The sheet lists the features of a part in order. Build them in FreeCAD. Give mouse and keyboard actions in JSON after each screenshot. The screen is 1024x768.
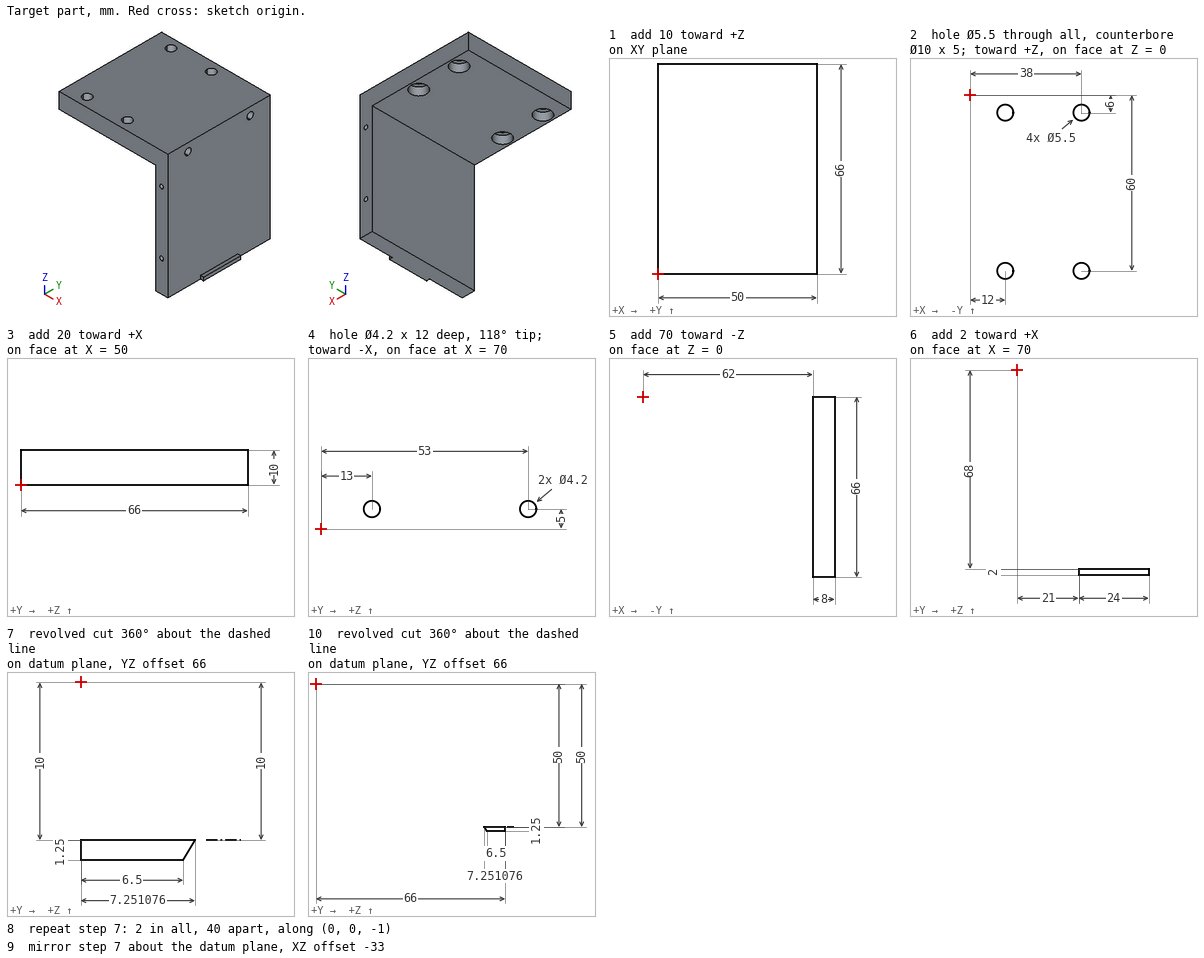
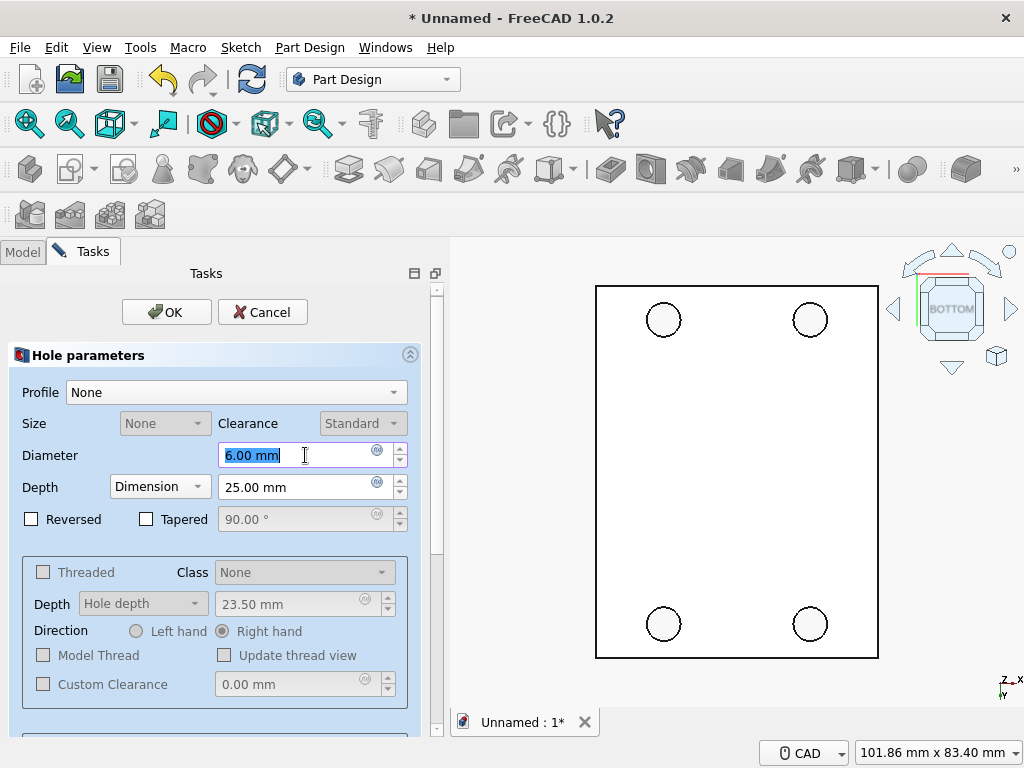
{"action": "type", "text": "5.5"}
{"action": "key", "text": "Tab"}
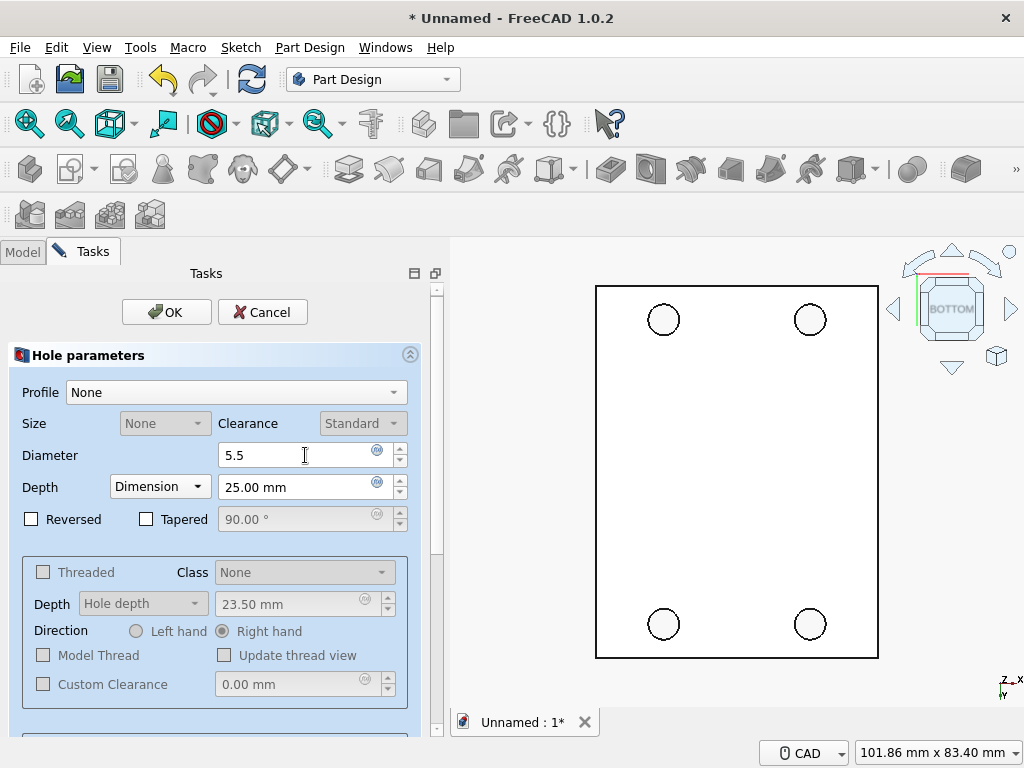
{"action": "left_click", "coordinate": [161, 486]}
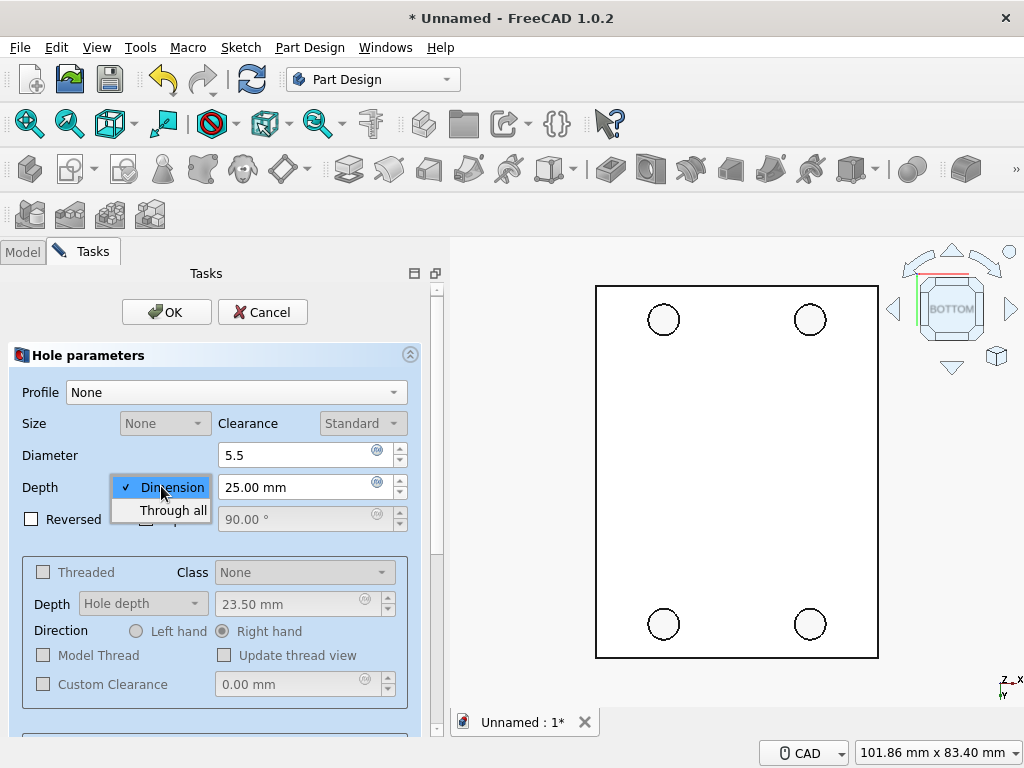
{"action": "left_click", "coordinate": [160, 510]}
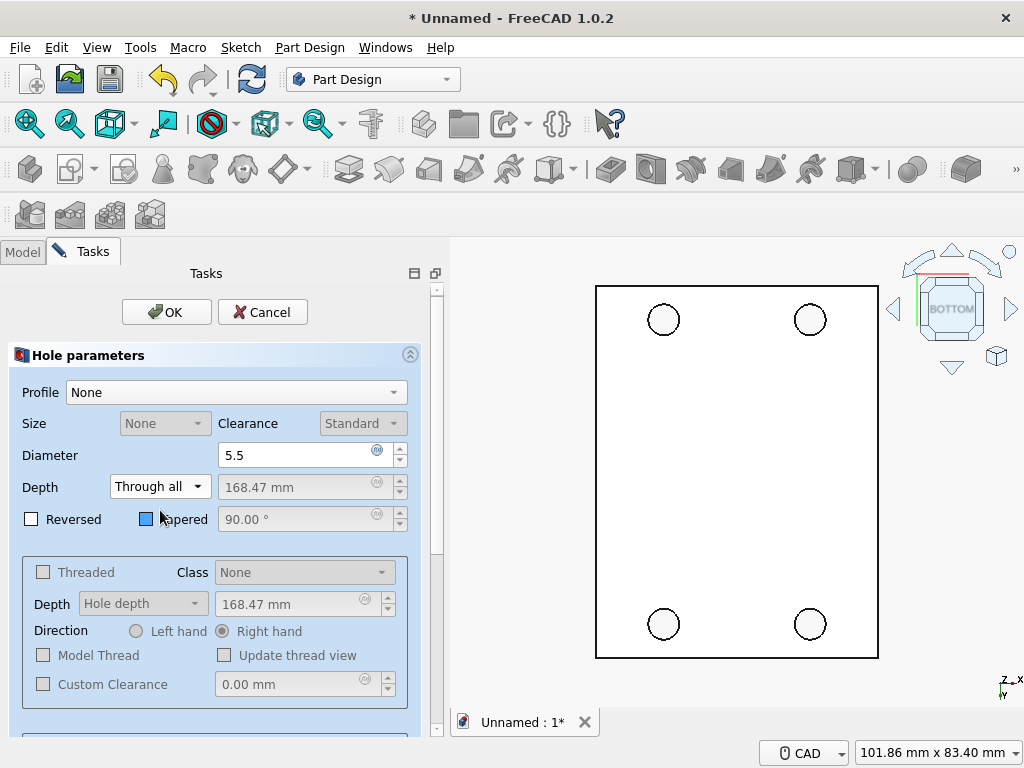
{"action": "scroll", "coordinate": [437, 510], "scroll_direction": "down", "scroll_amount": 2}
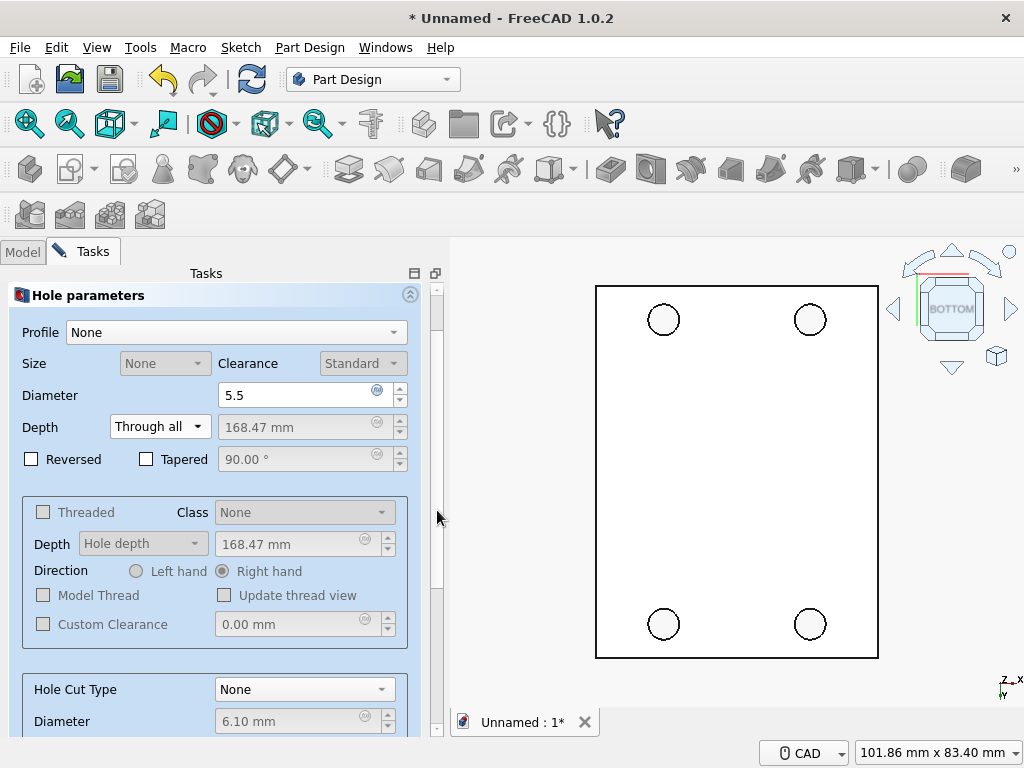
{"action": "left_click", "coordinate": [306, 630]}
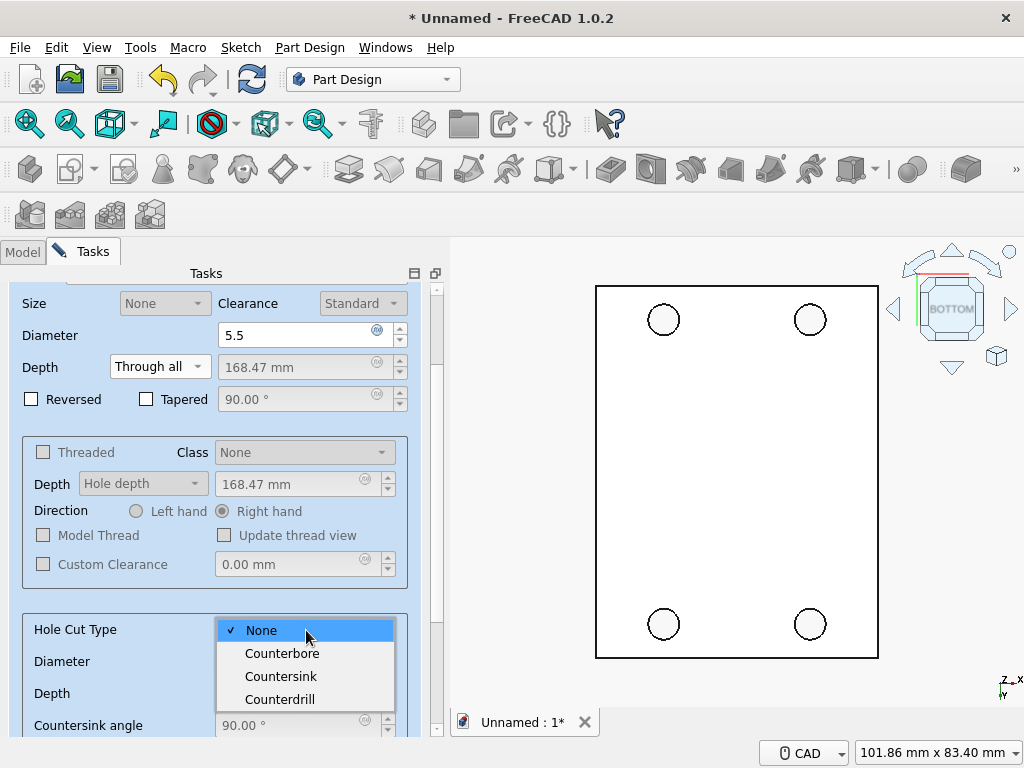
{"action": "left_click", "coordinate": [304, 654]}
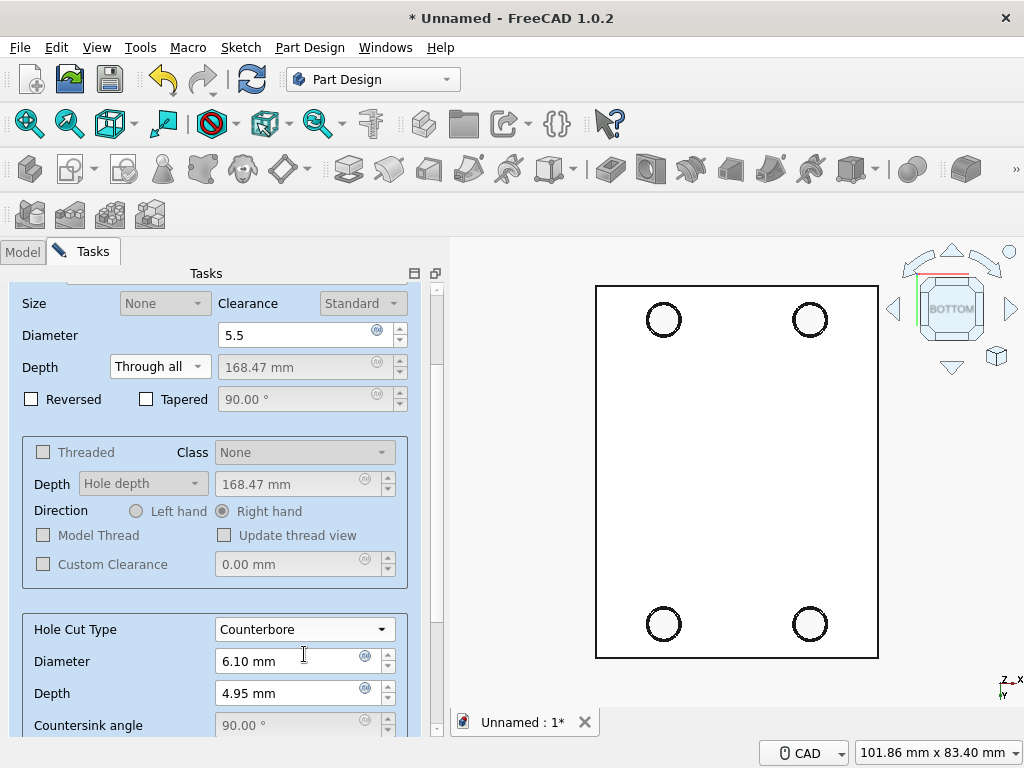
{"action": "triple_click", "coordinate": [298, 661]}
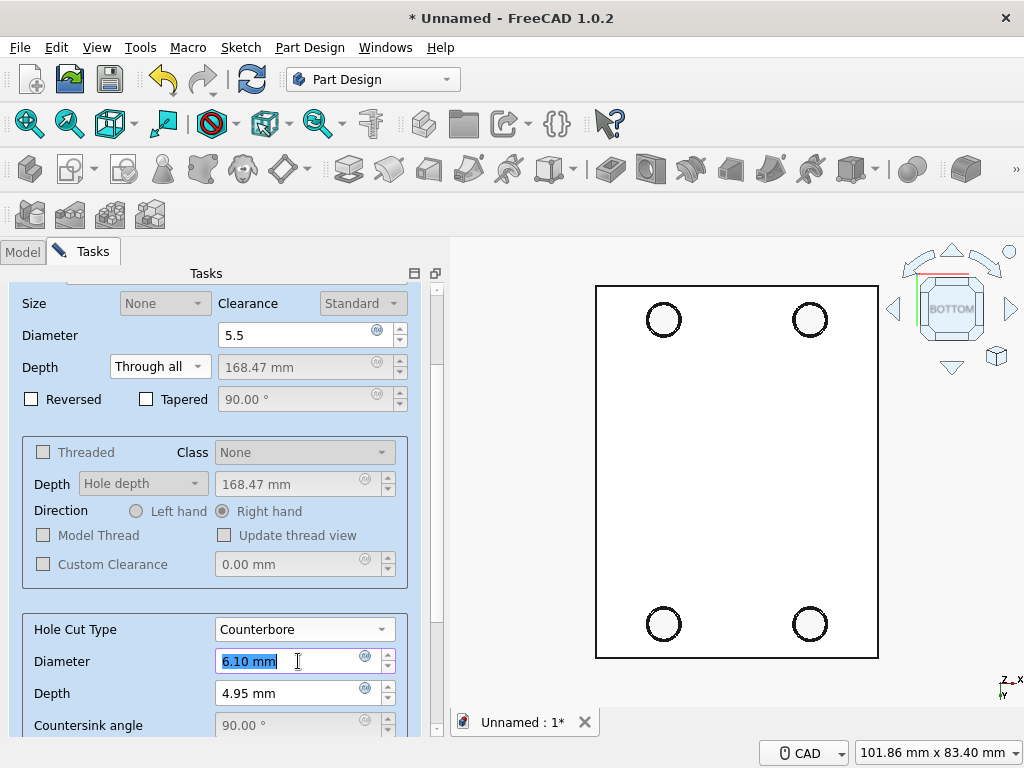
{"action": "type", "text": "10"}
{"action": "key", "text": "Tab"}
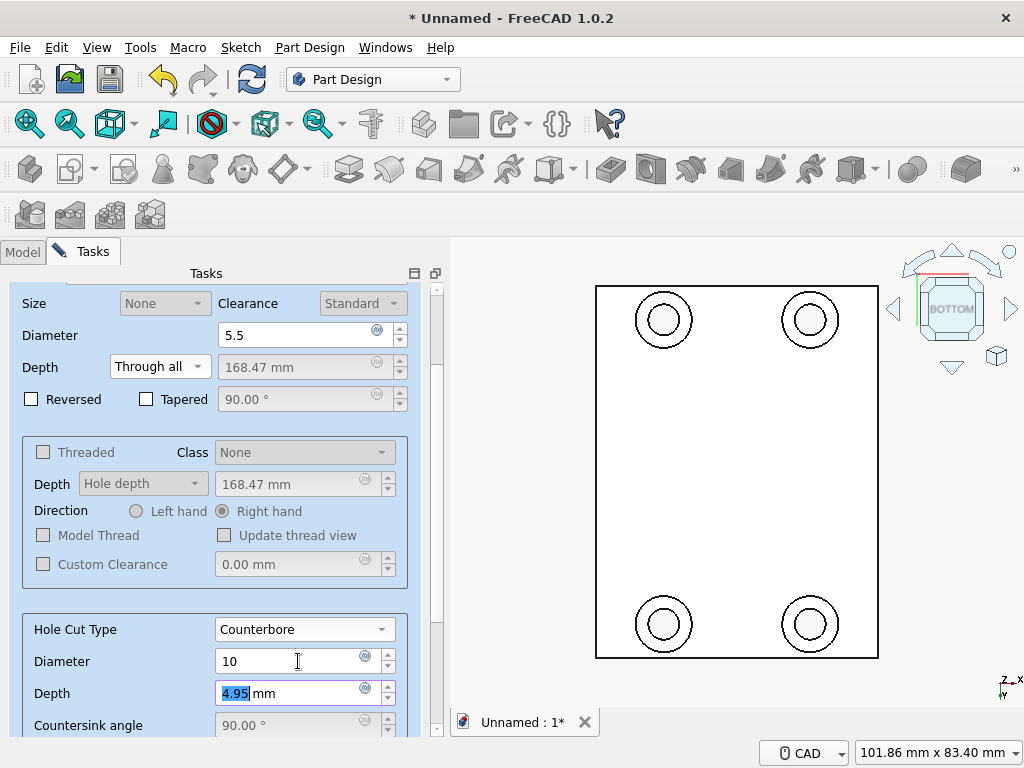
{"action": "type", "text": "5"}
{"action": "key", "text": "Tab"}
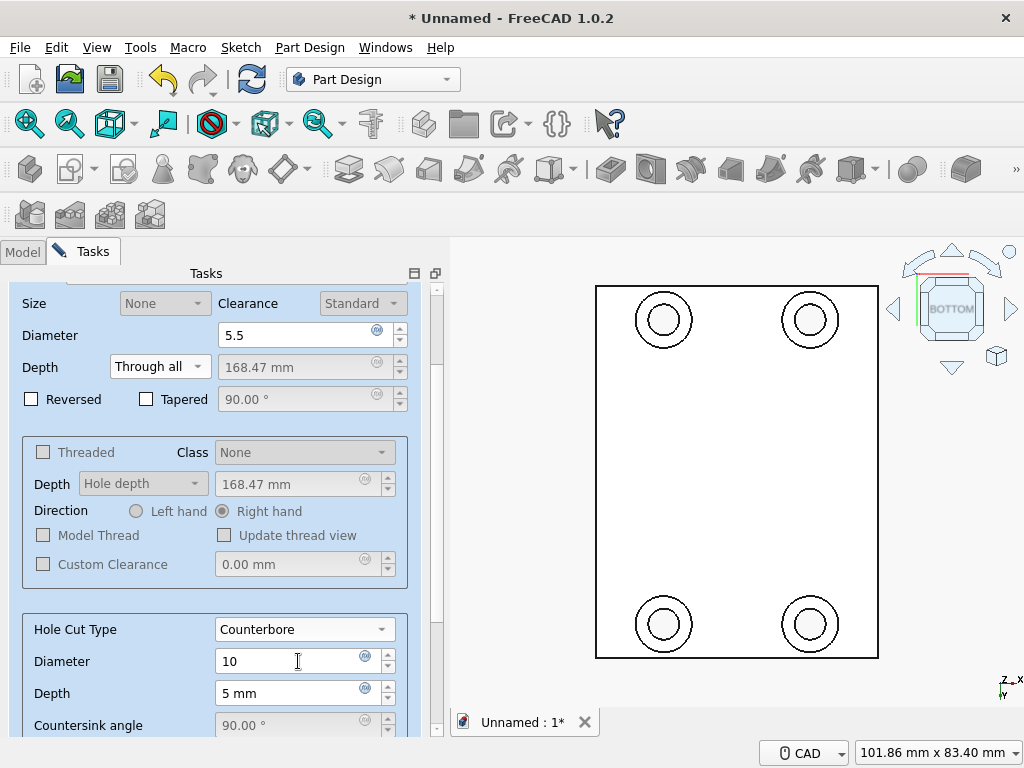
{"action": "scroll", "coordinate": [437, 510], "scroll_direction": "up", "scroll_amount": 3}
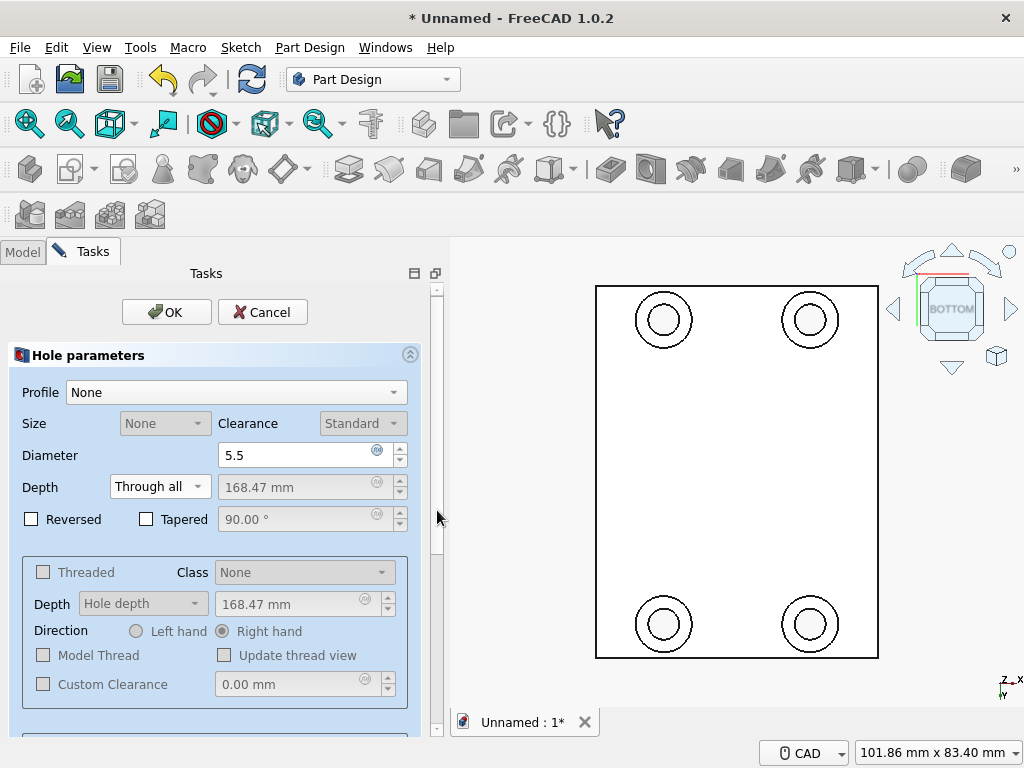
{"action": "left_click", "coordinate": [167, 312]}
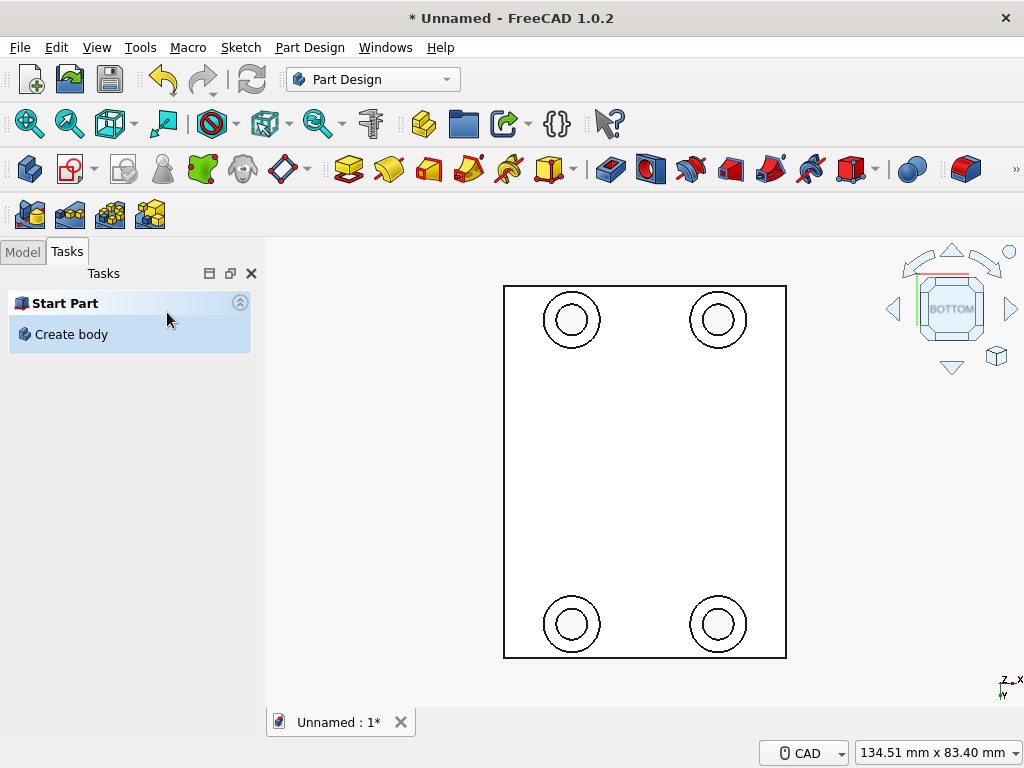
{"action": "key", "text": "0"}